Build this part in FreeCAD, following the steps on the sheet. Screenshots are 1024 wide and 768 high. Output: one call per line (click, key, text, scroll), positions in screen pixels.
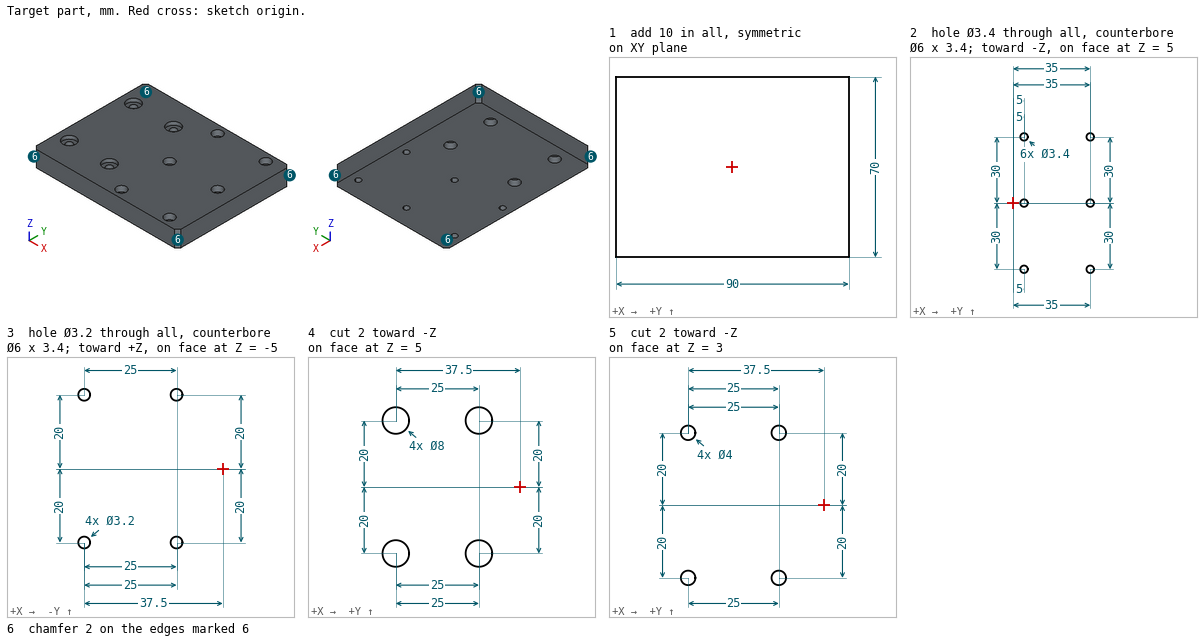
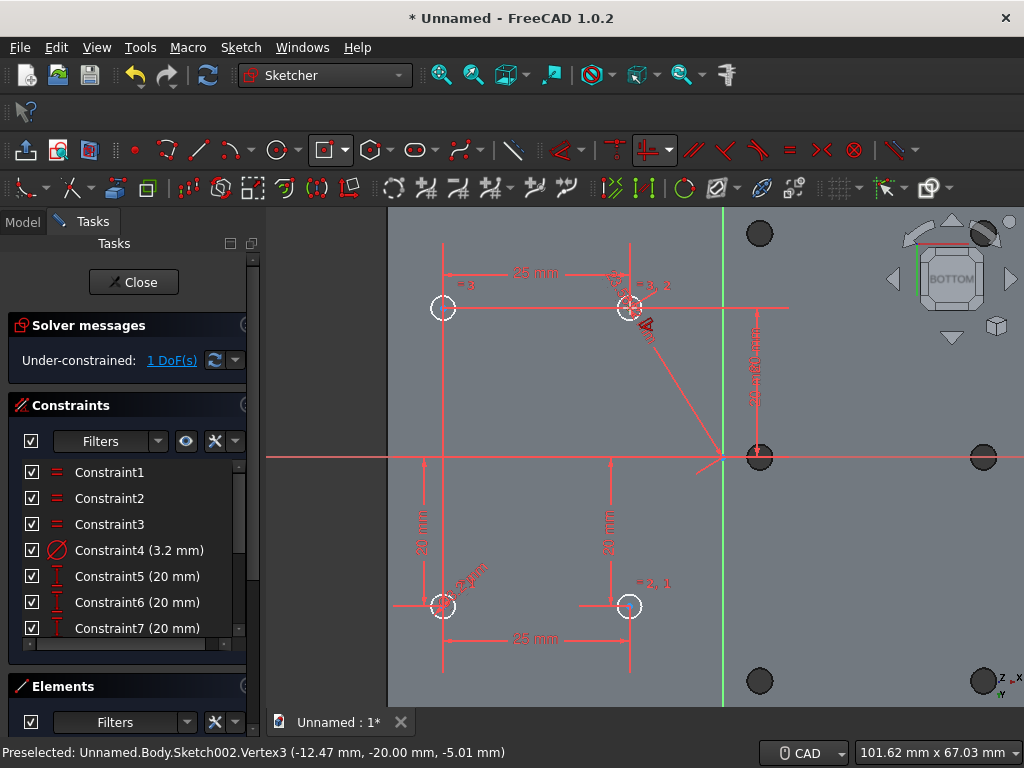
click(443, 308)
click(536, 342)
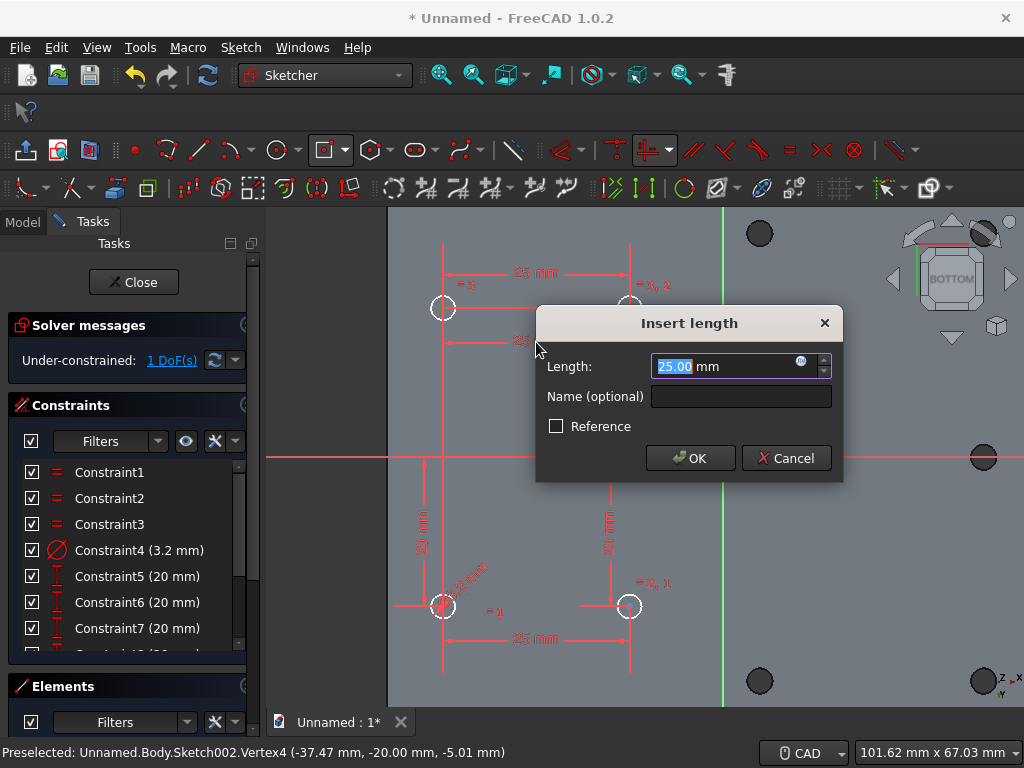
text(25)
key(Return)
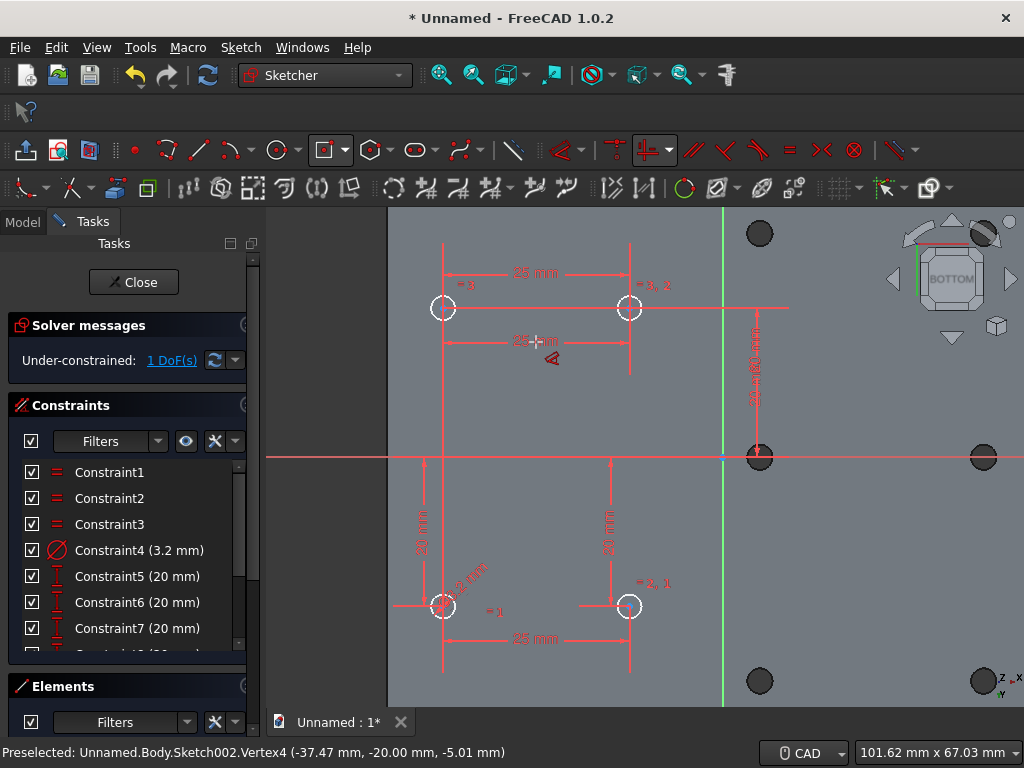
click(443, 606)
click(647, 640)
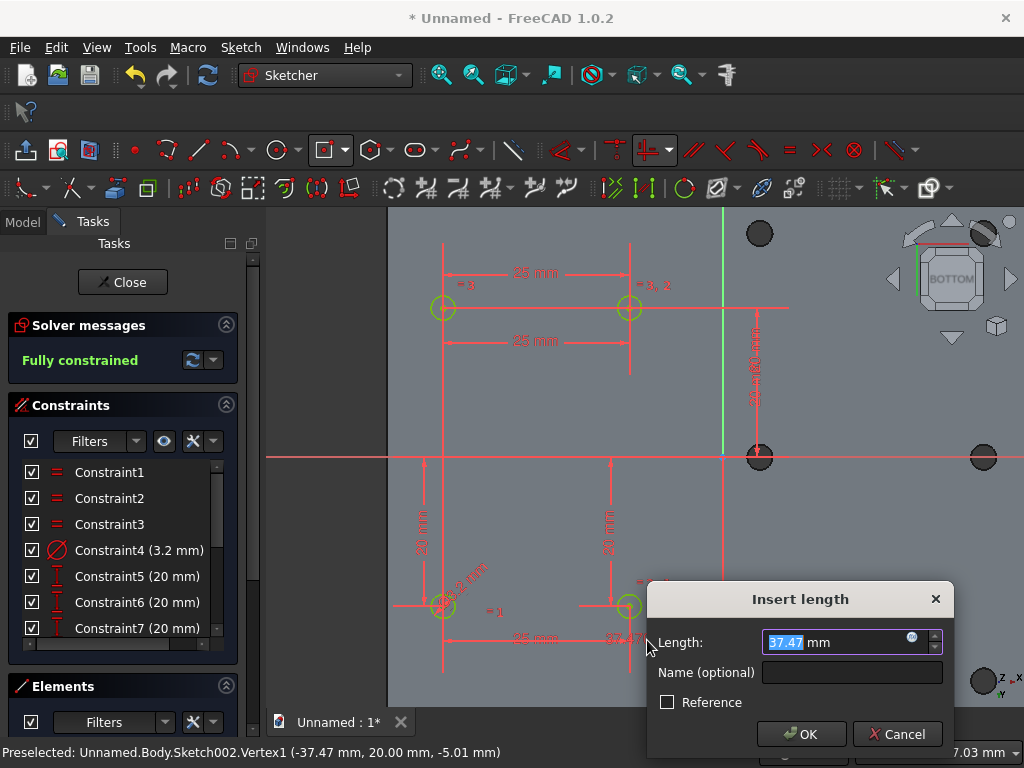
text(37.5)
key(Return)
key(Escape)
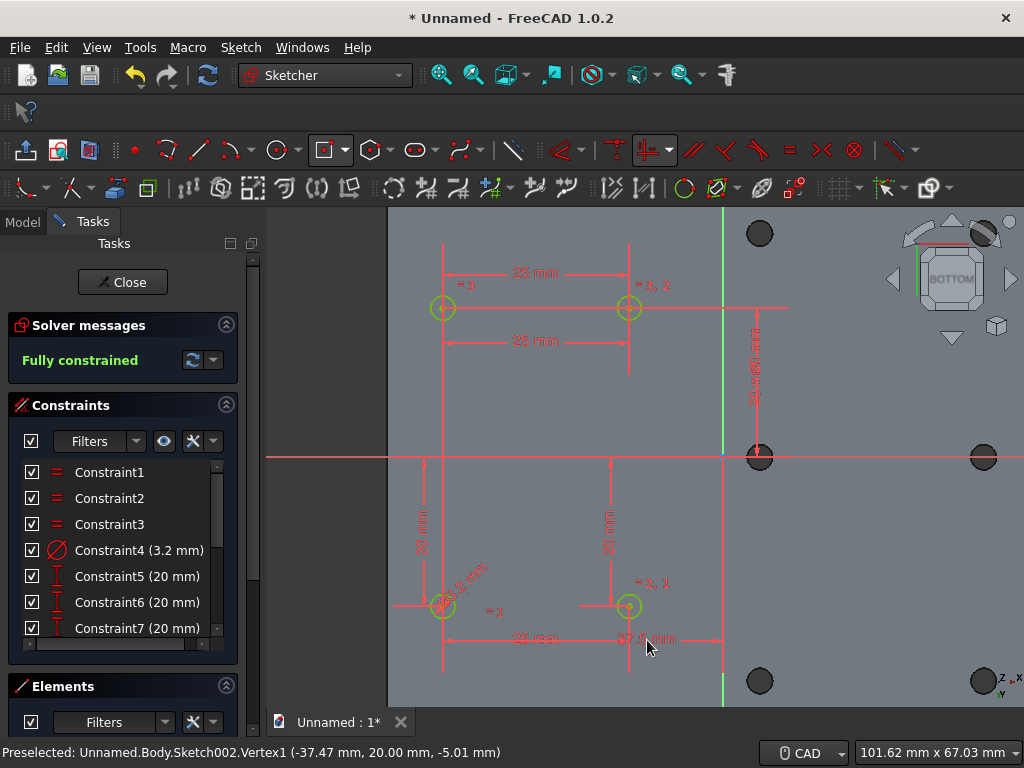
click(123, 282)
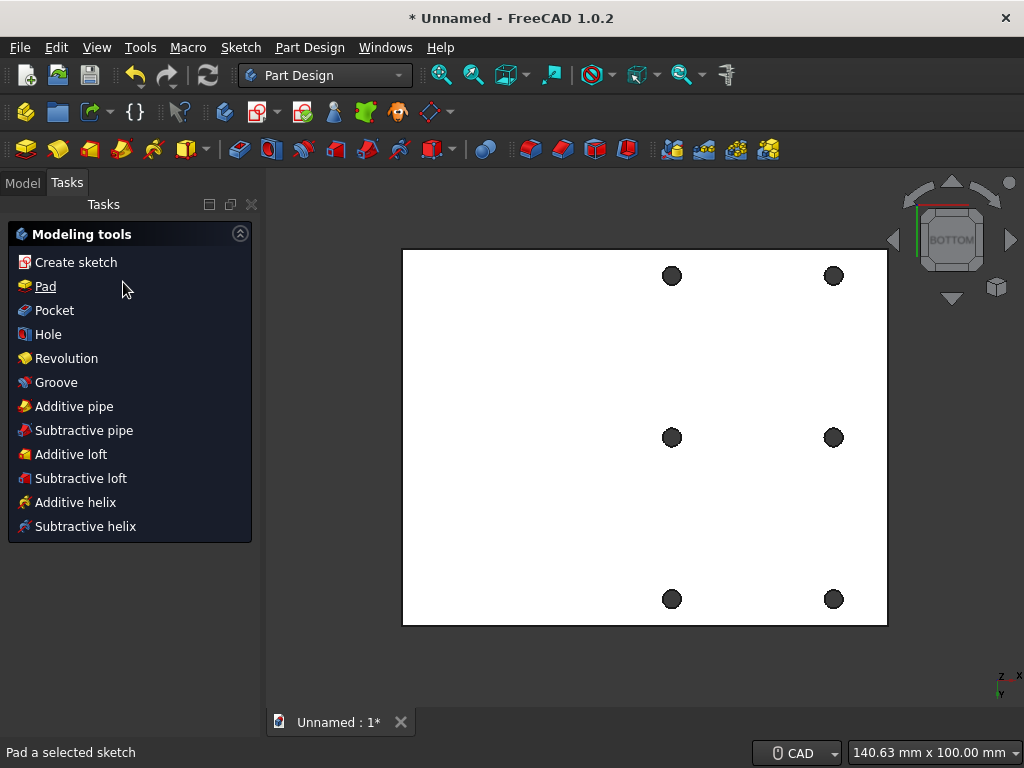
click(272, 150)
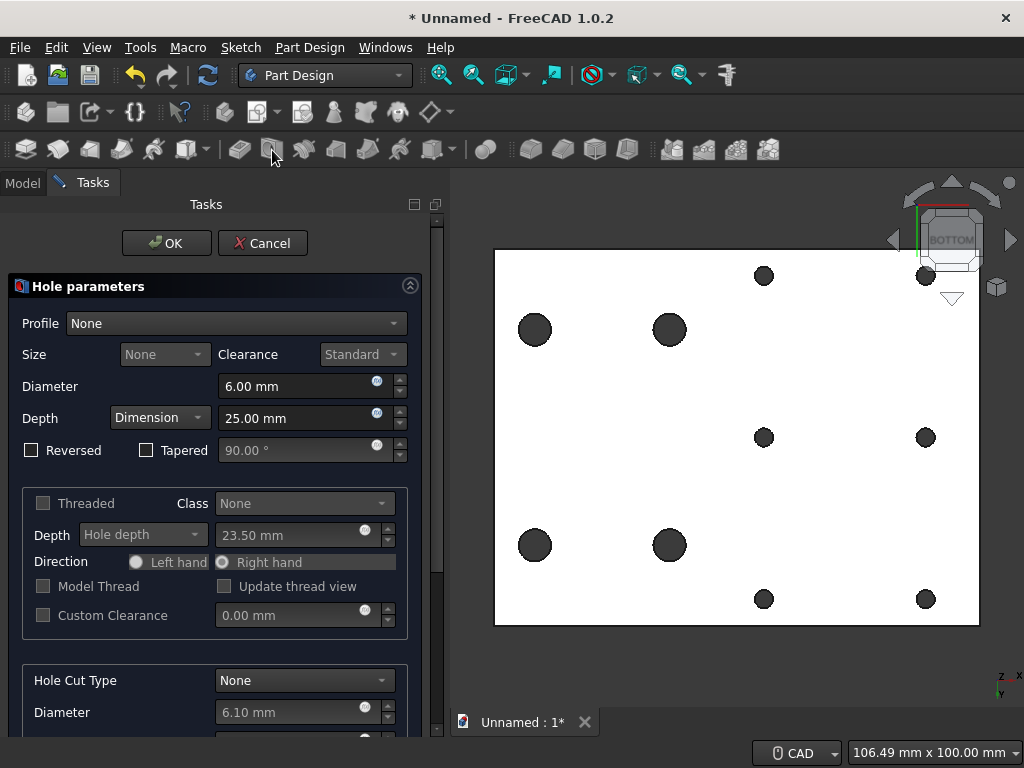
triple_click(305, 386)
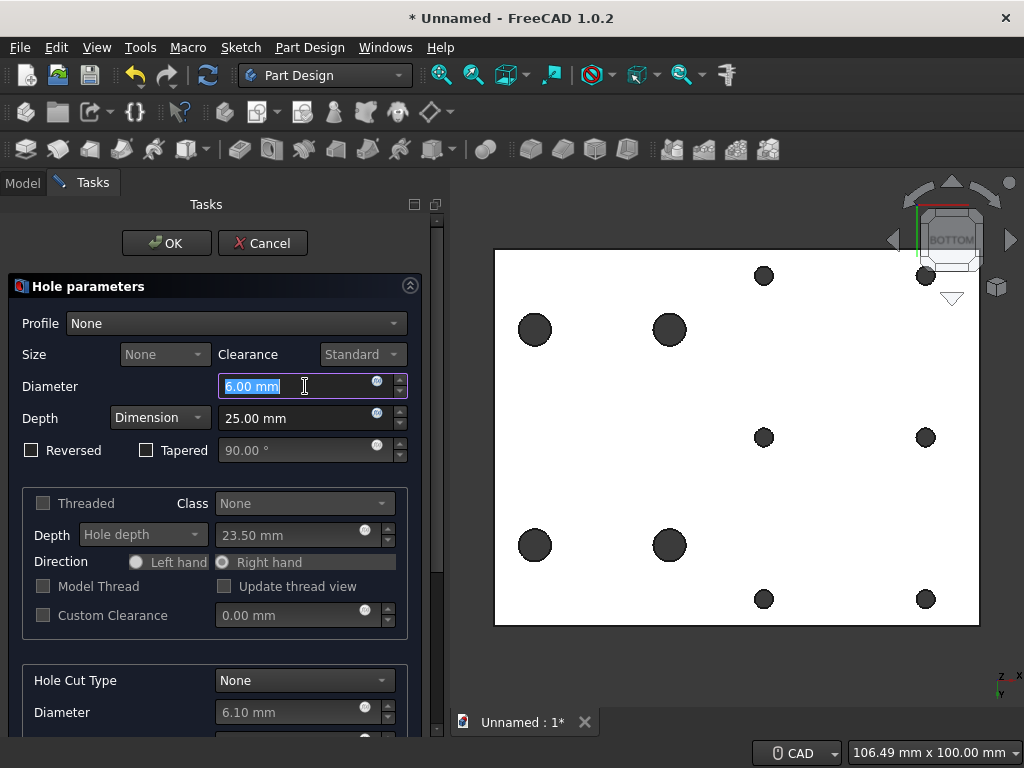
text(3.2)
key(Tab)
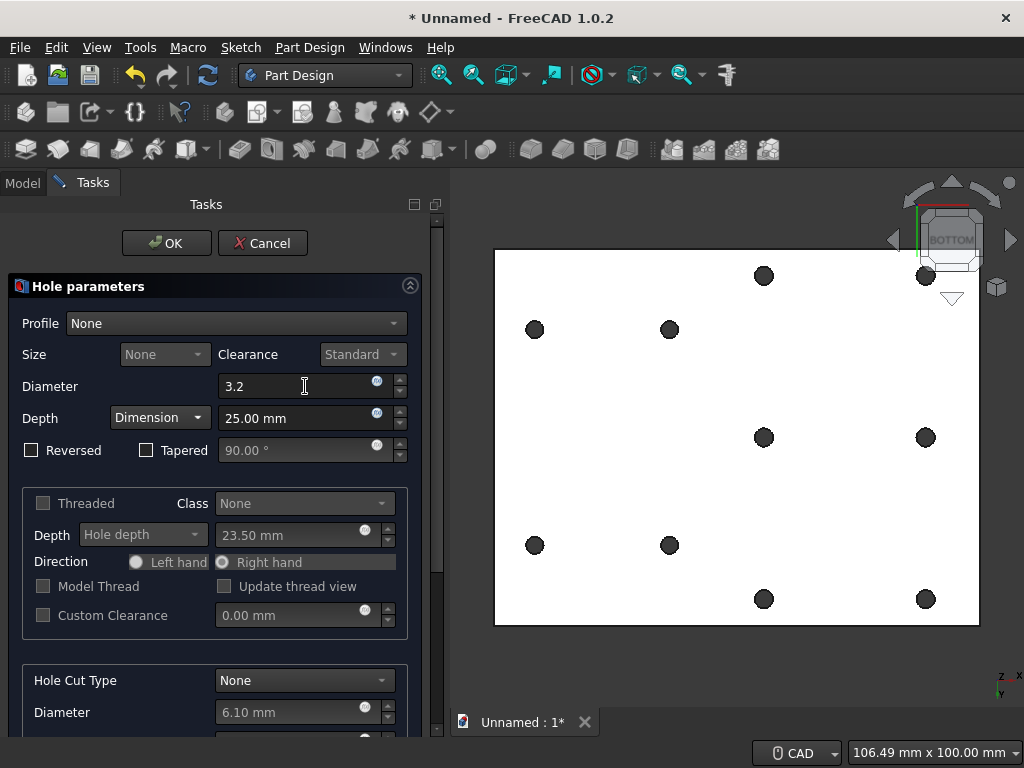
click(161, 418)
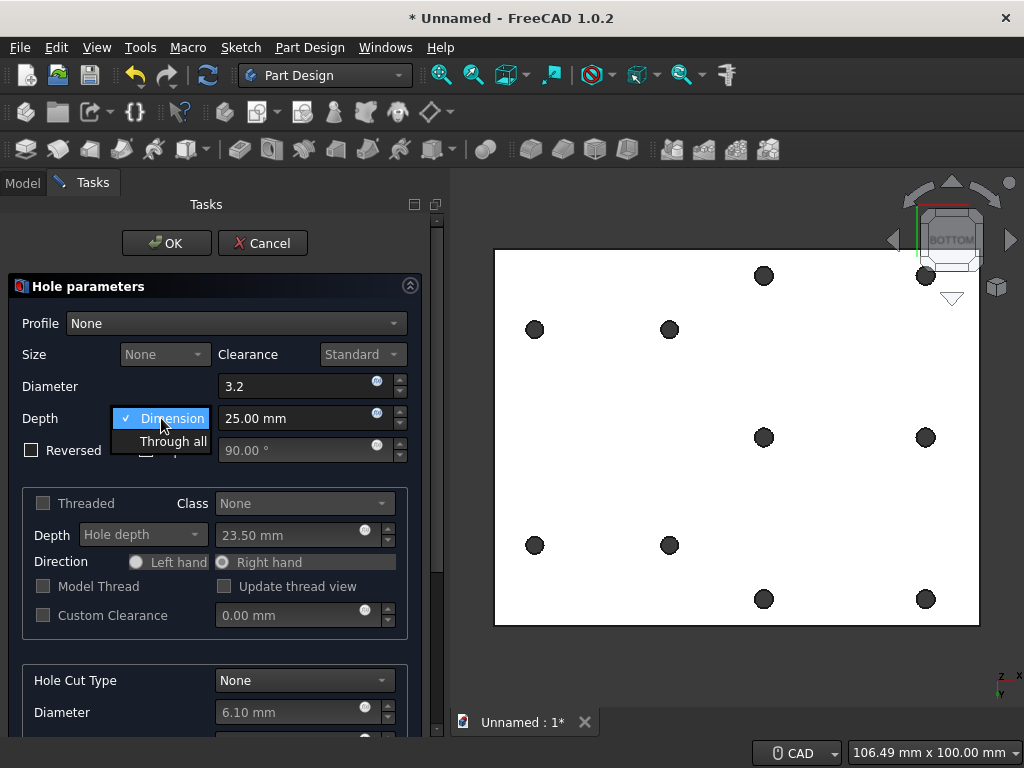
click(160, 442)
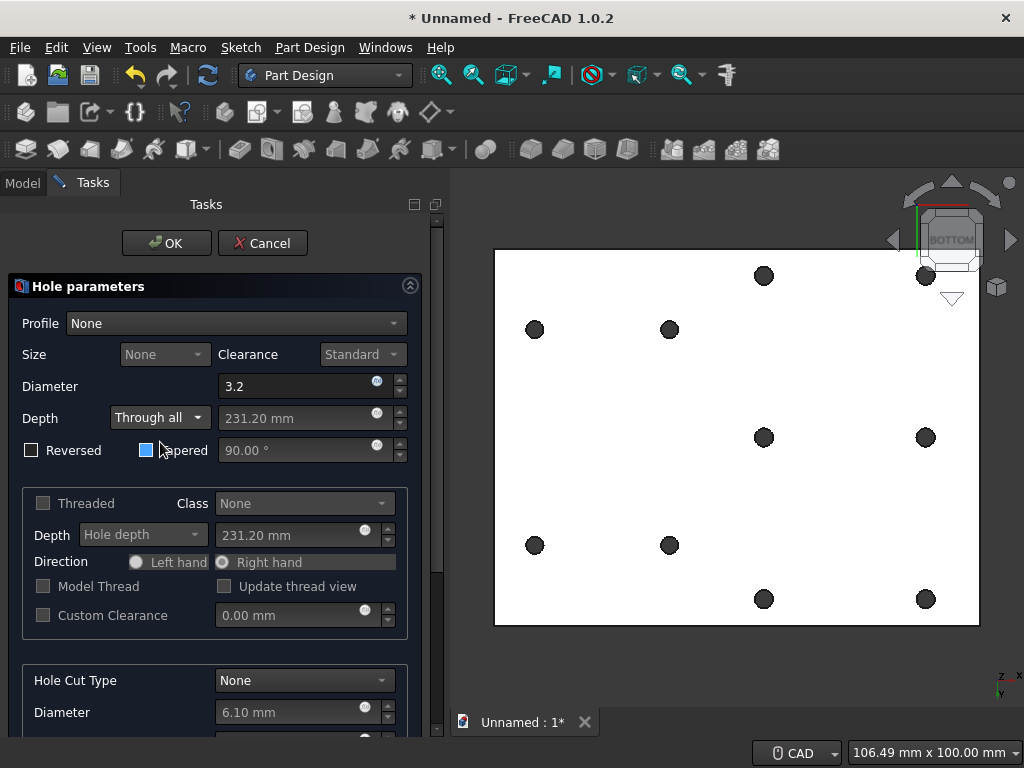
click(306, 680)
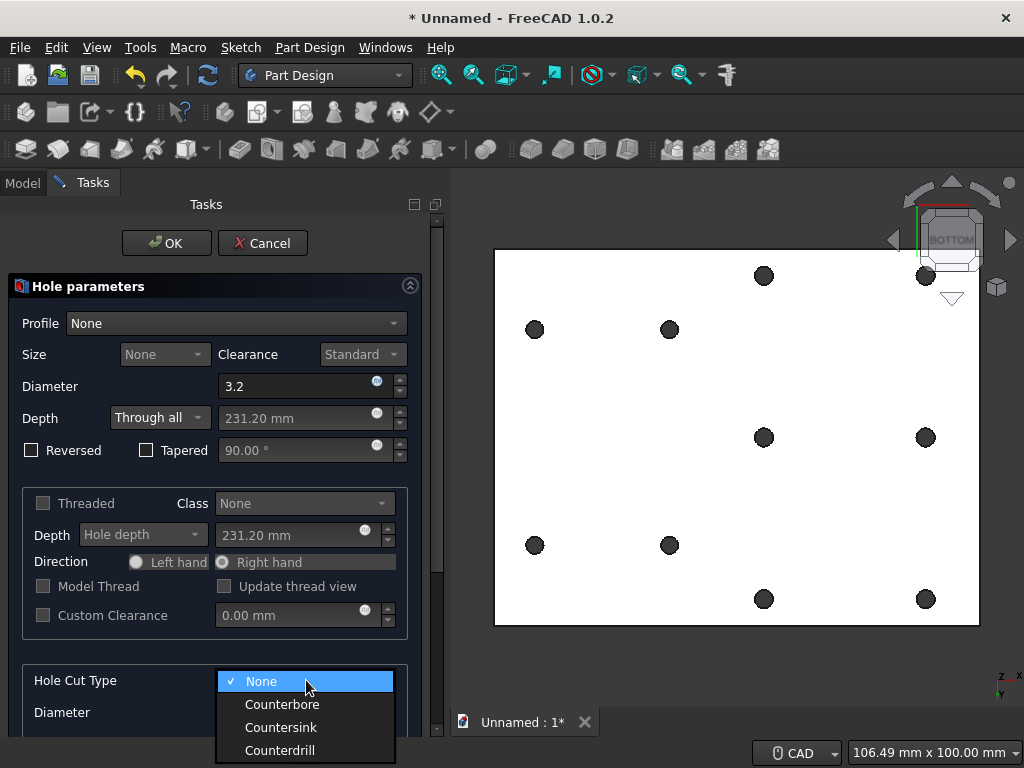
click(304, 704)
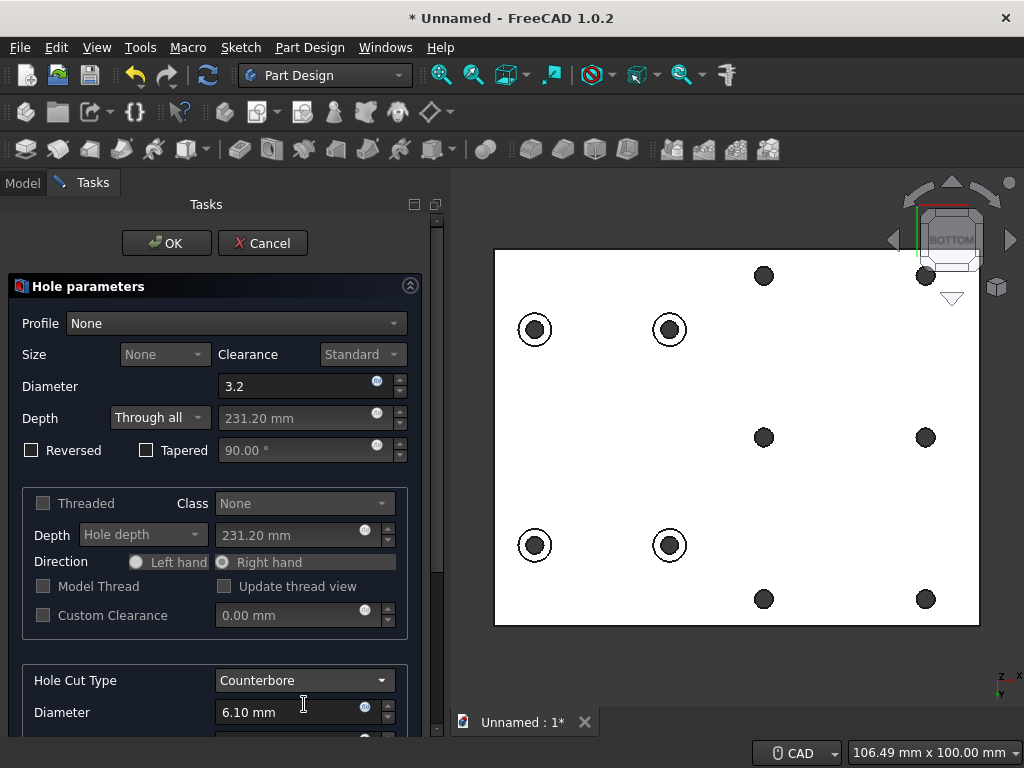
triple_click(298, 712)